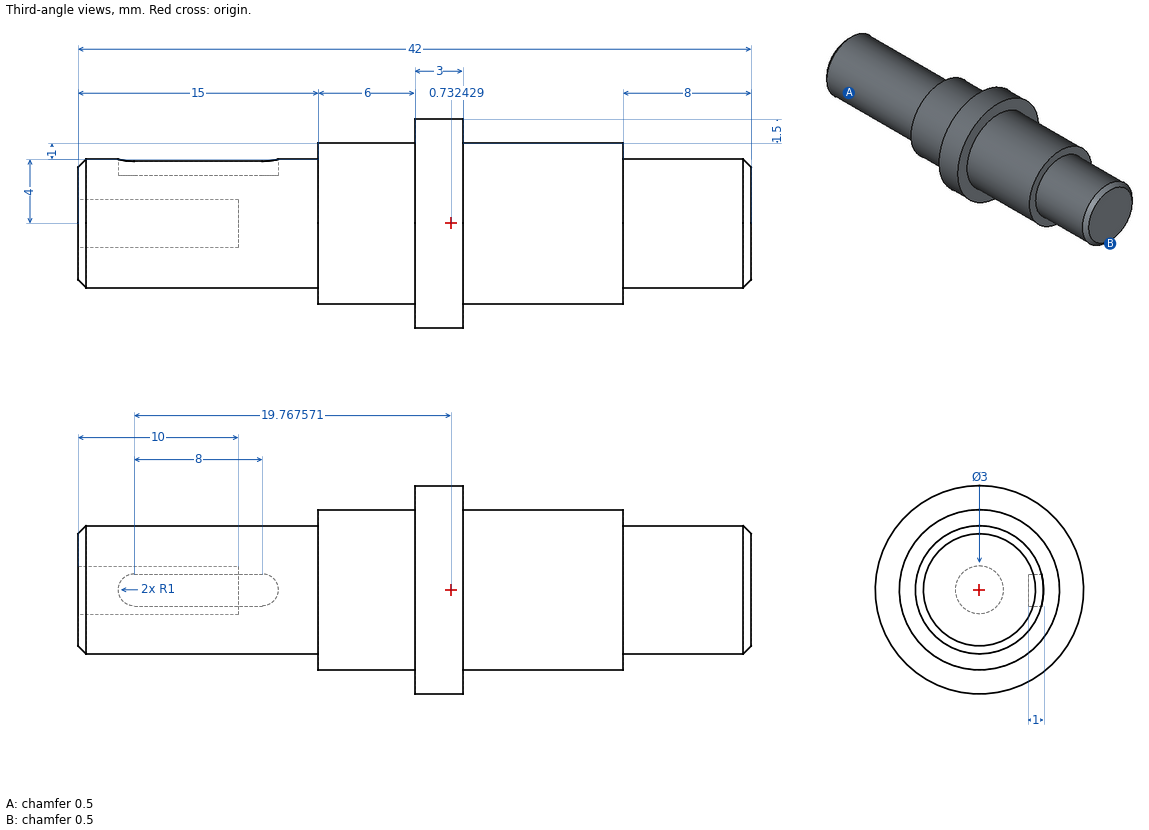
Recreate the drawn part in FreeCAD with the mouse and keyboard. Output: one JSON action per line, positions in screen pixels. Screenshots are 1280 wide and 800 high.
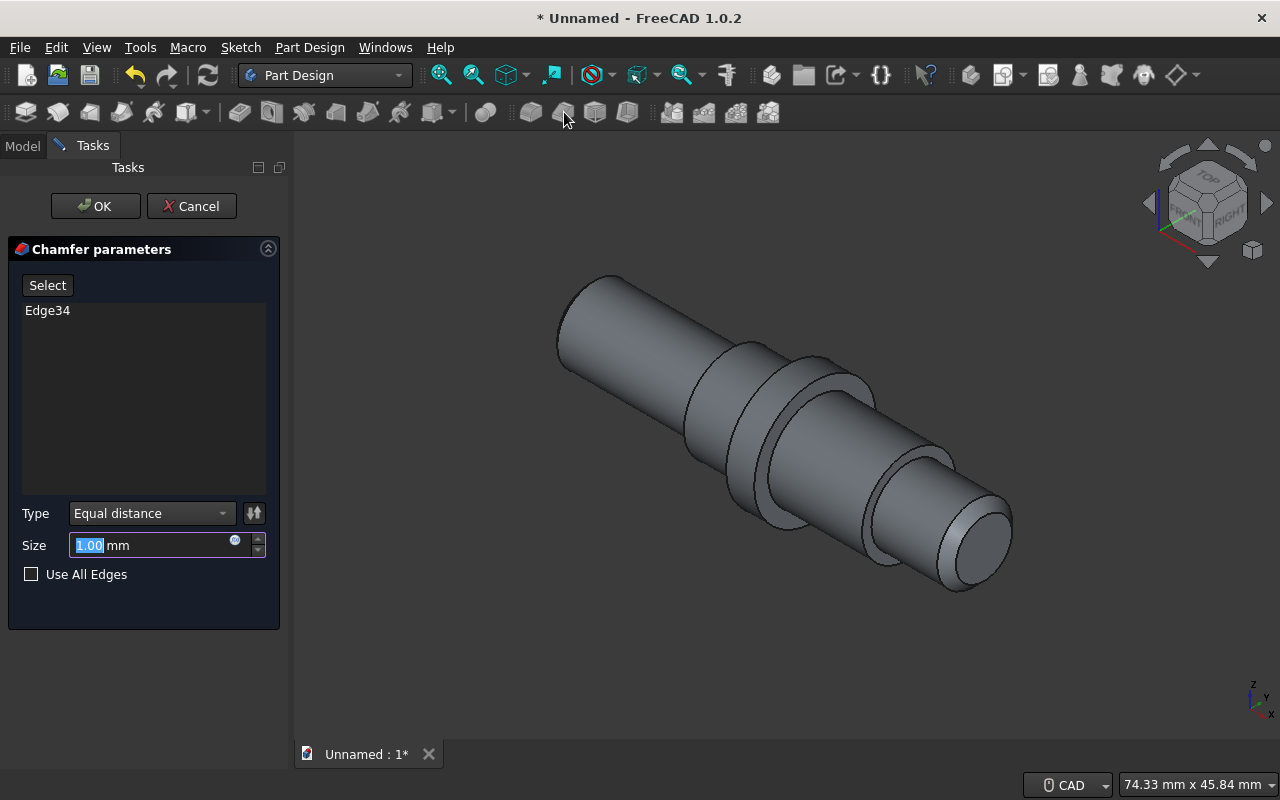
{"action": "type", "text": "0.5"}
{"action": "key", "text": "Tab"}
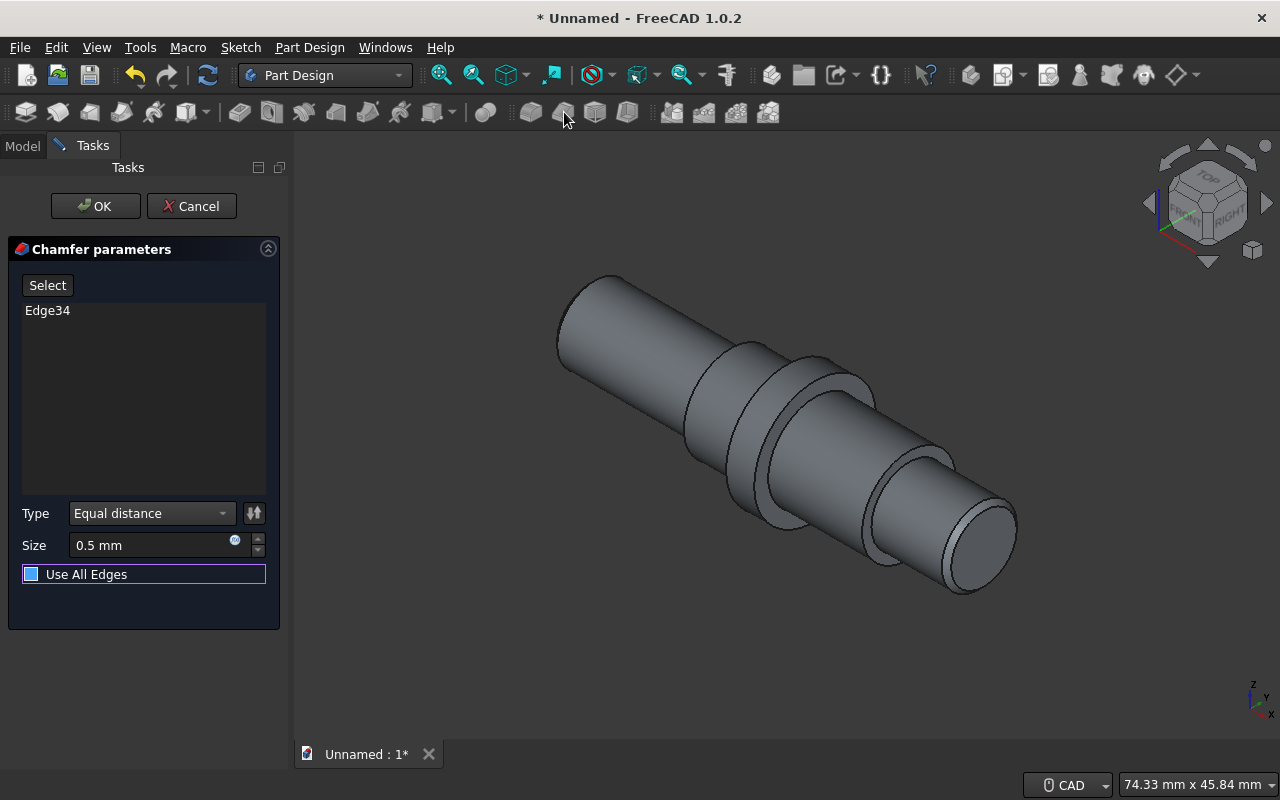
{"action": "left_click", "coordinate": [96, 206]}